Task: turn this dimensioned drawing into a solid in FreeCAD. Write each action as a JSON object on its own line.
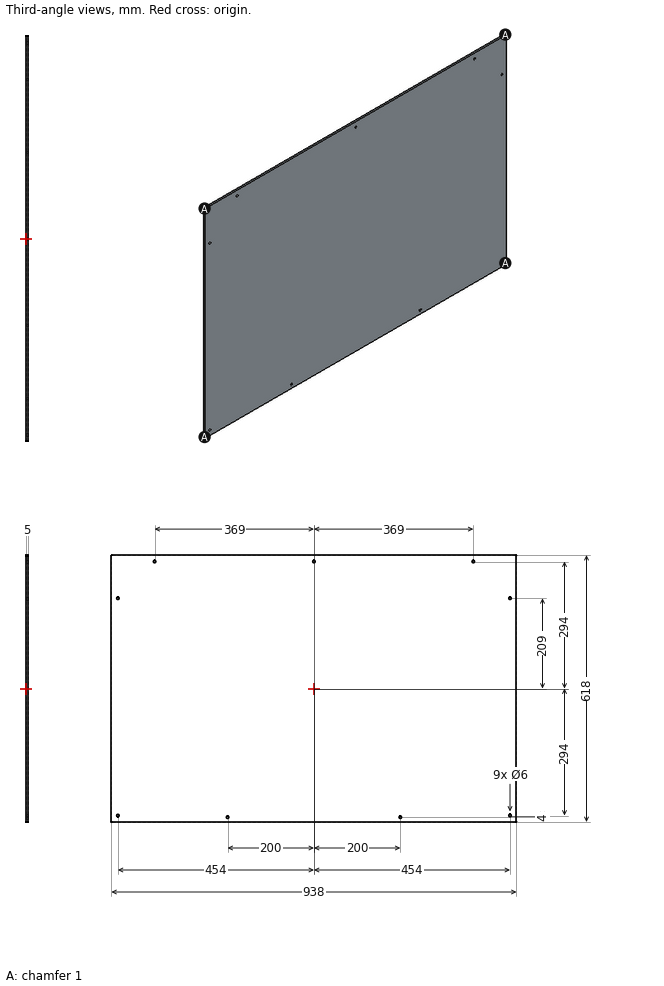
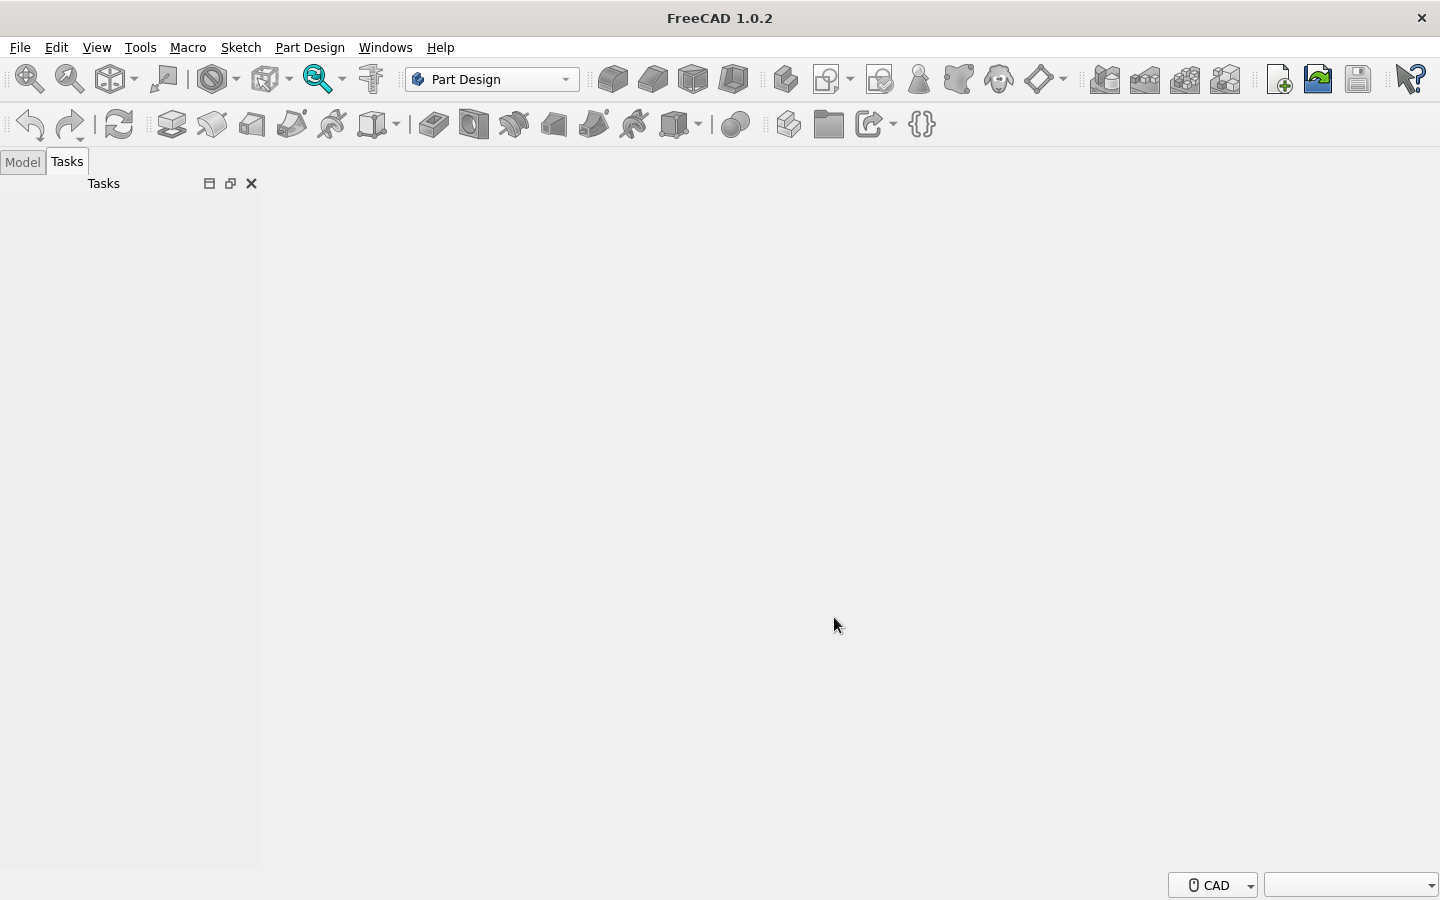
{"action": "left_click", "coordinate": [1278, 80]}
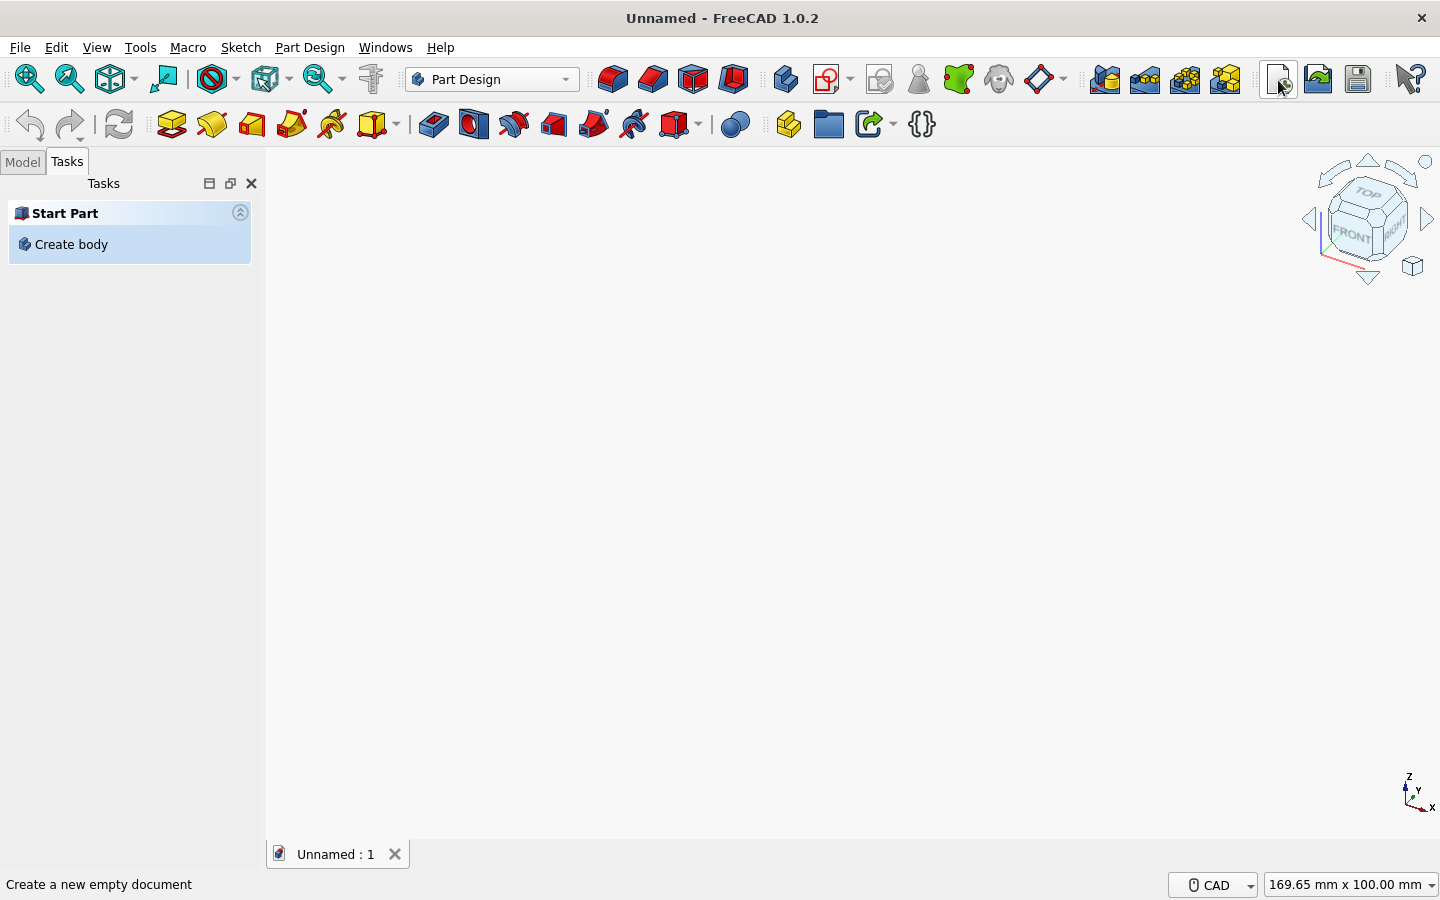
{"action": "left_click", "coordinate": [826, 80]}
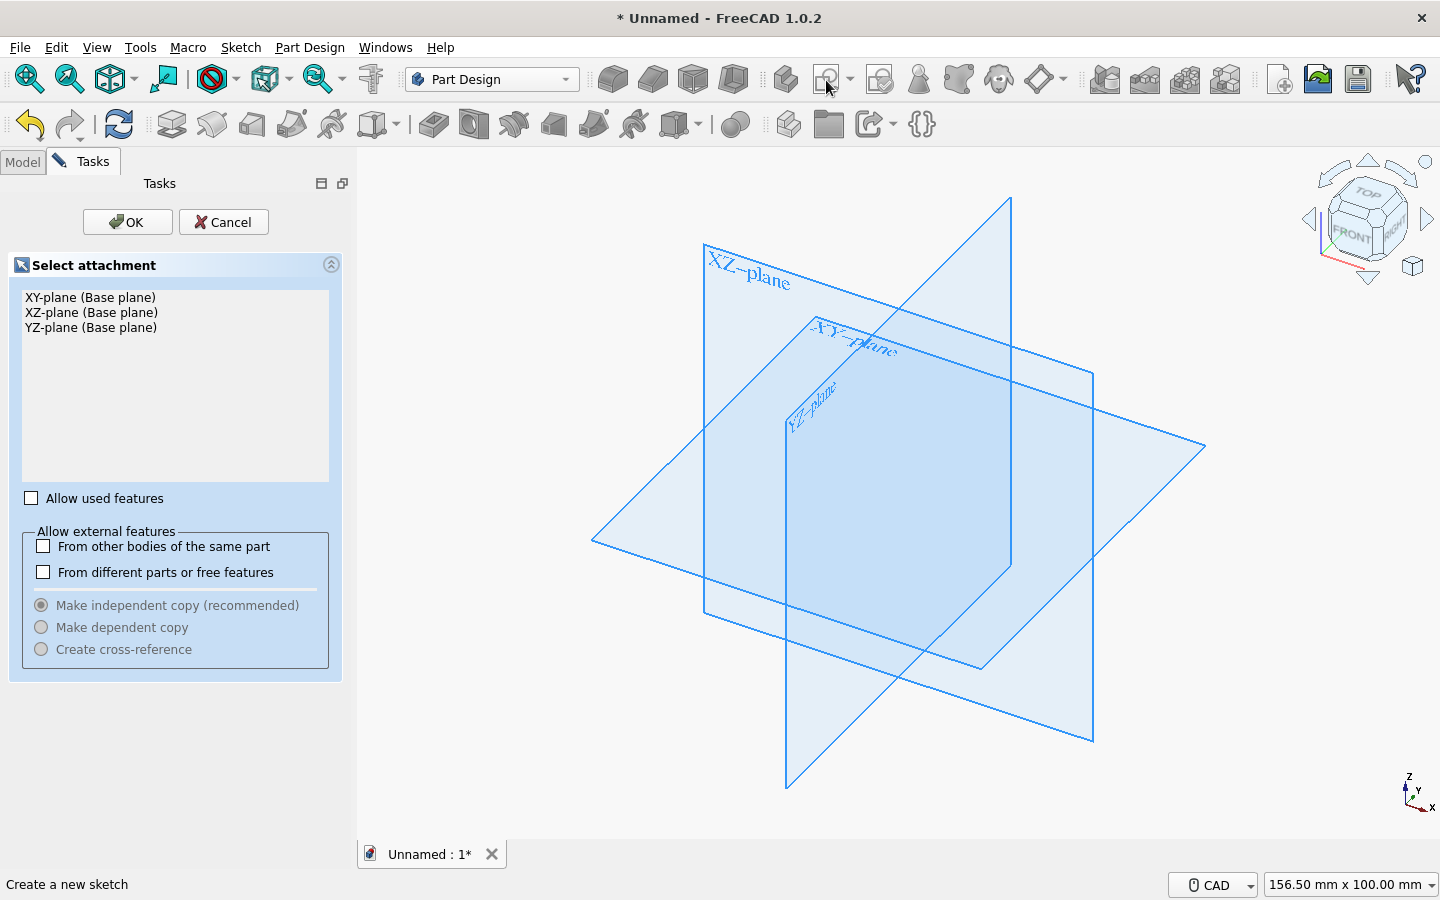
{"action": "left_click", "coordinate": [82, 328]}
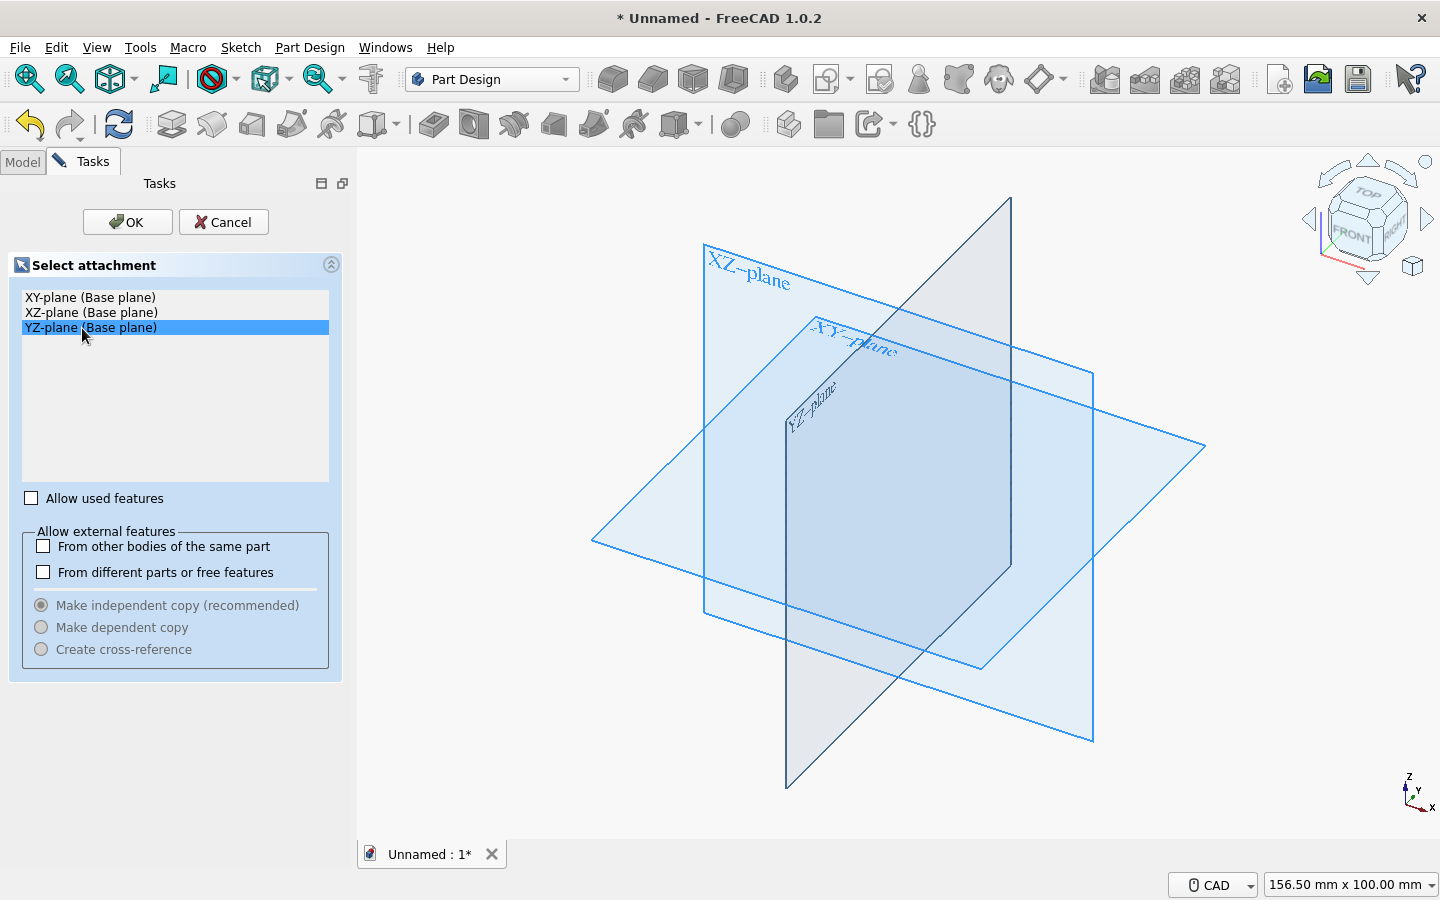
{"action": "left_click", "coordinate": [128, 222]}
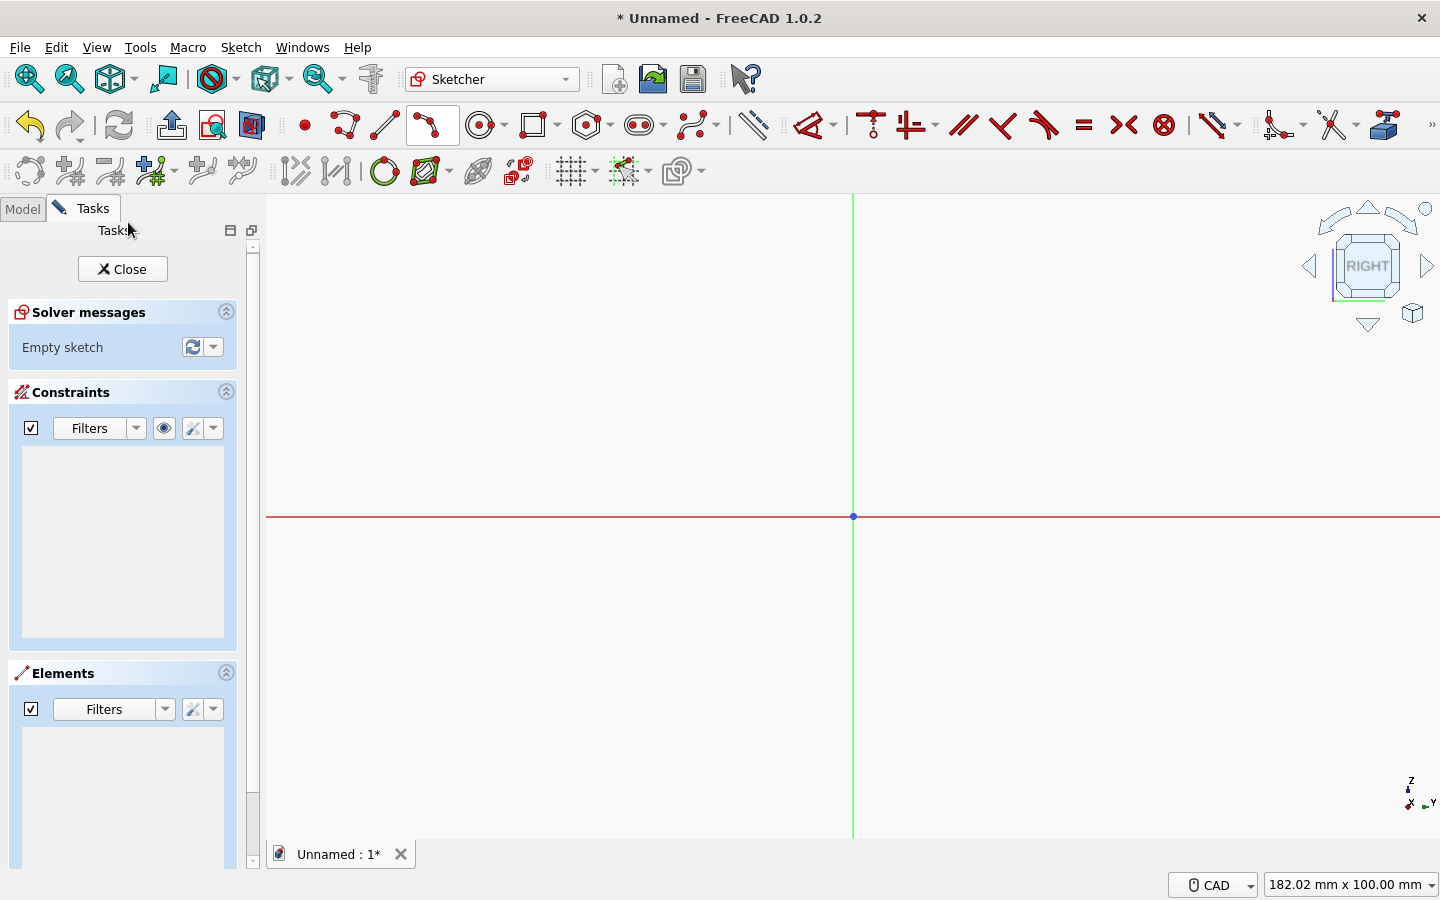
{"action": "scroll", "coordinate": [776, 516], "scroll_direction": "down", "scroll_amount": 11}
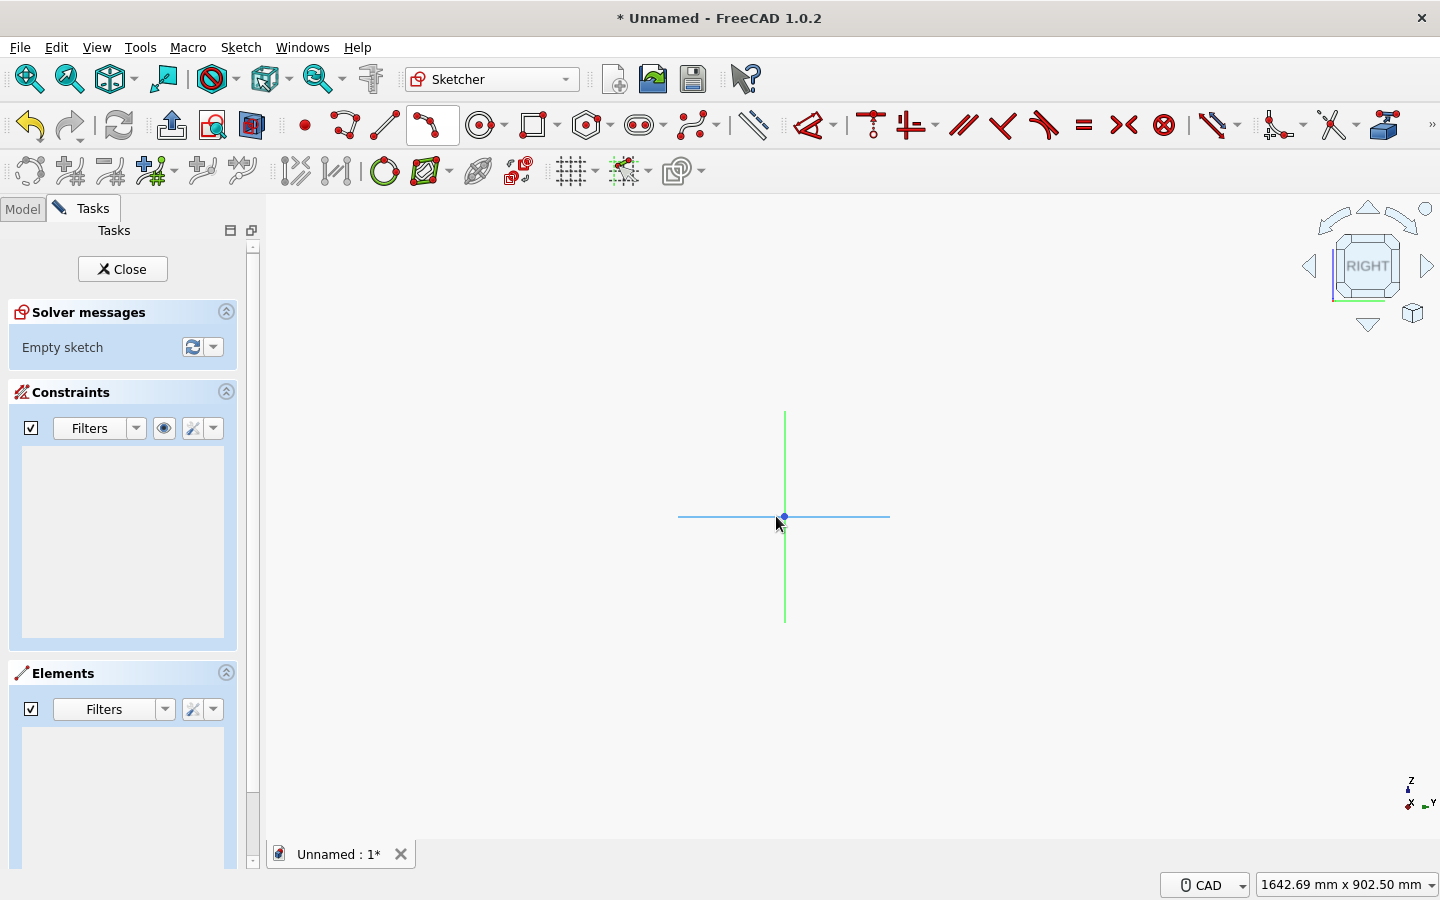
{"action": "left_click", "coordinate": [560, 126]}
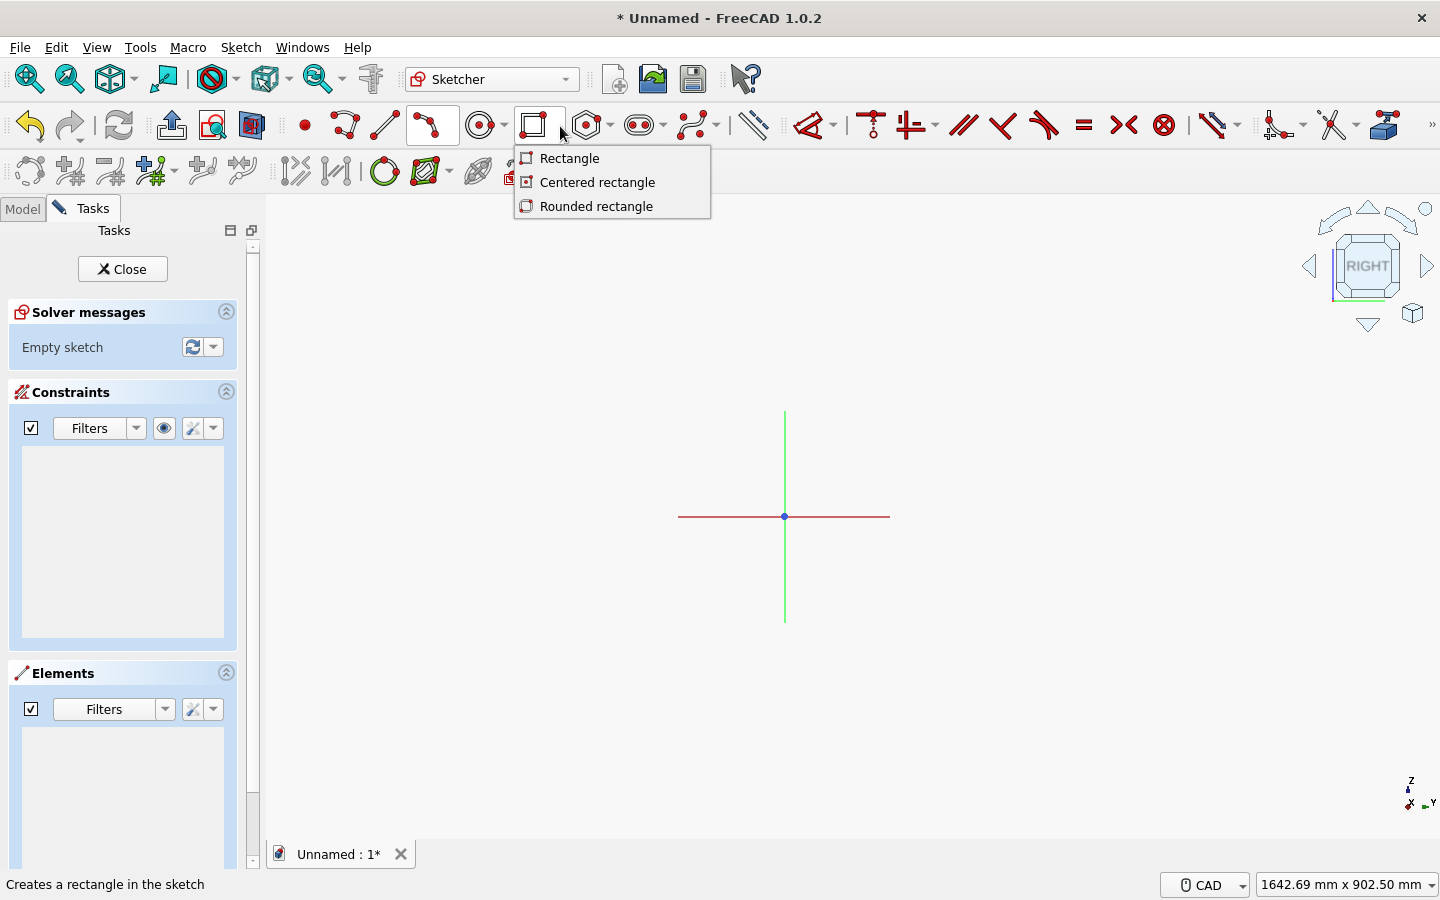
{"action": "left_click", "coordinate": [612, 182]}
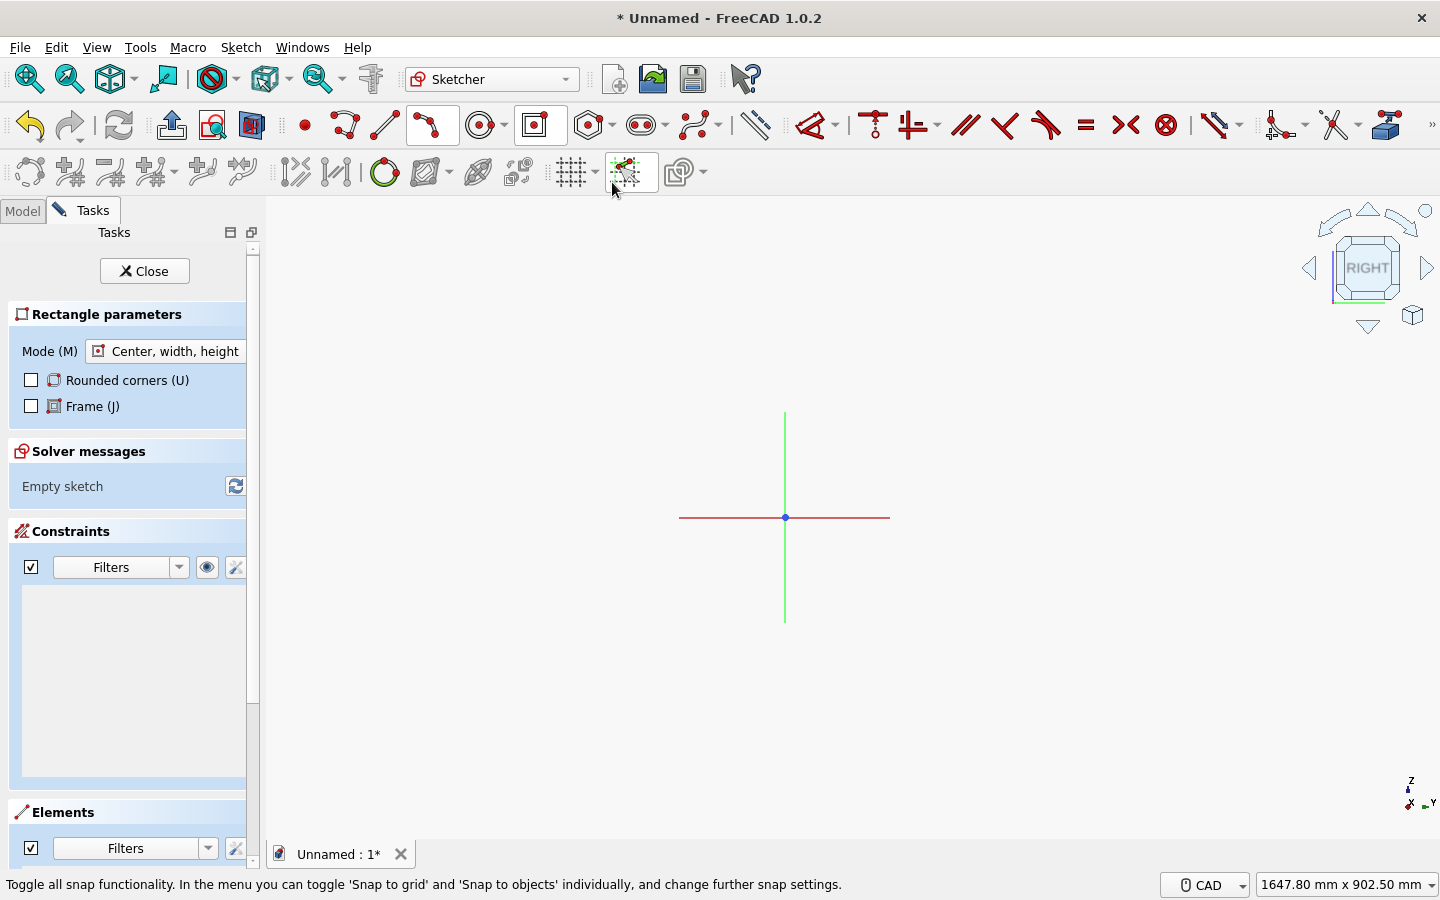
{"action": "left_click", "coordinate": [785, 518]}
{"action": "left_click", "coordinate": [1119, 297]}
{"action": "key", "text": "Escape"}